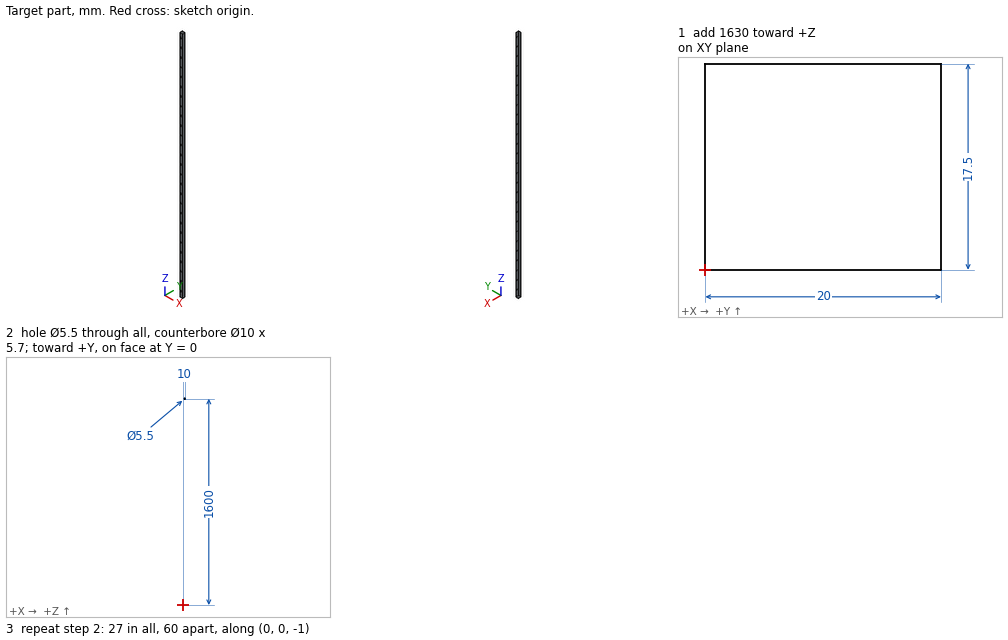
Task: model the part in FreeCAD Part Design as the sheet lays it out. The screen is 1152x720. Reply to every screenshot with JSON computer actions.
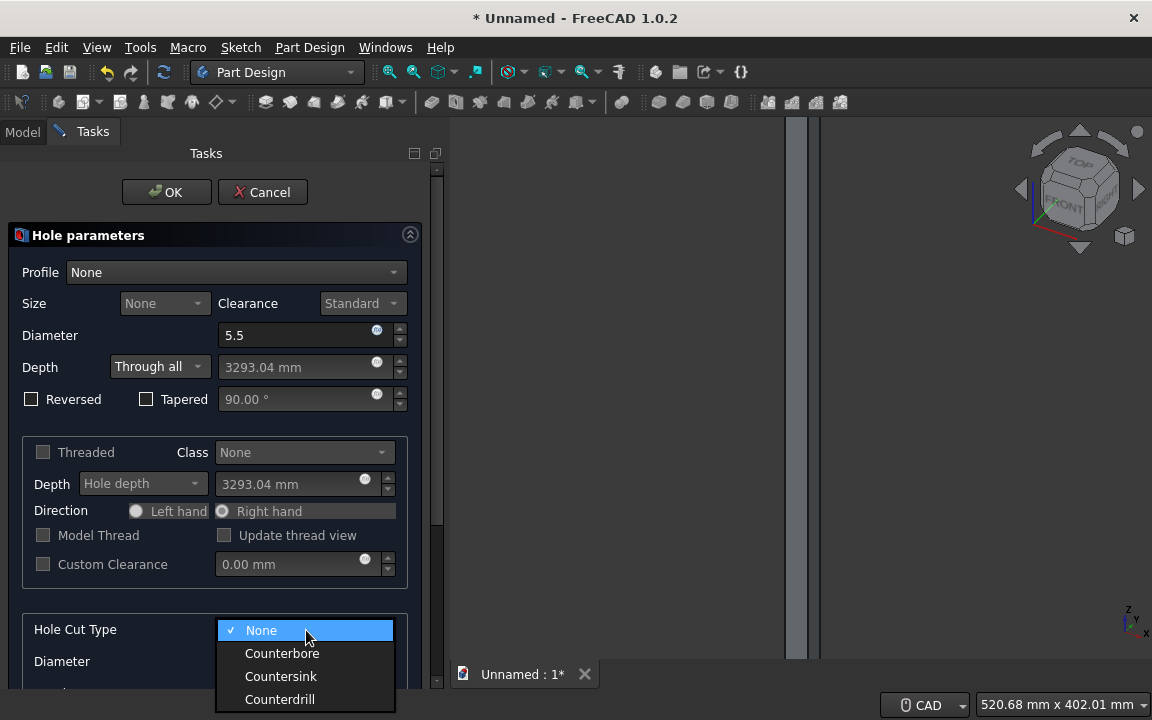
{"action": "left_click", "coordinate": [304, 654]}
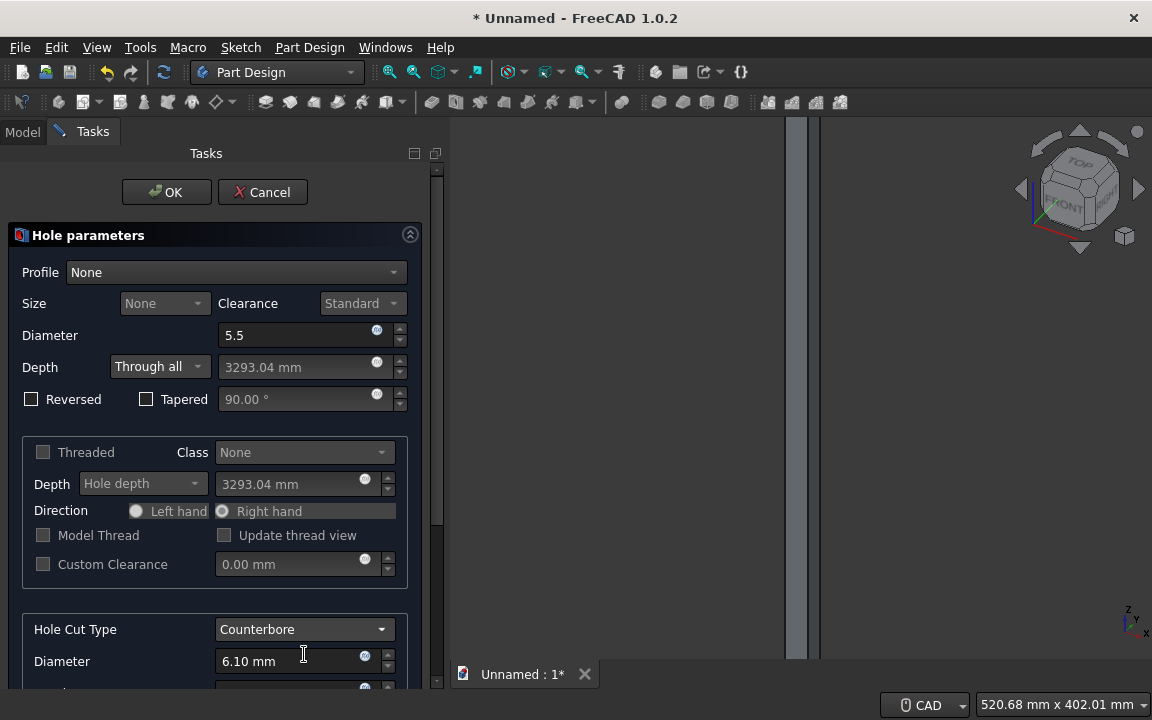
{"action": "triple_click", "coordinate": [298, 661]}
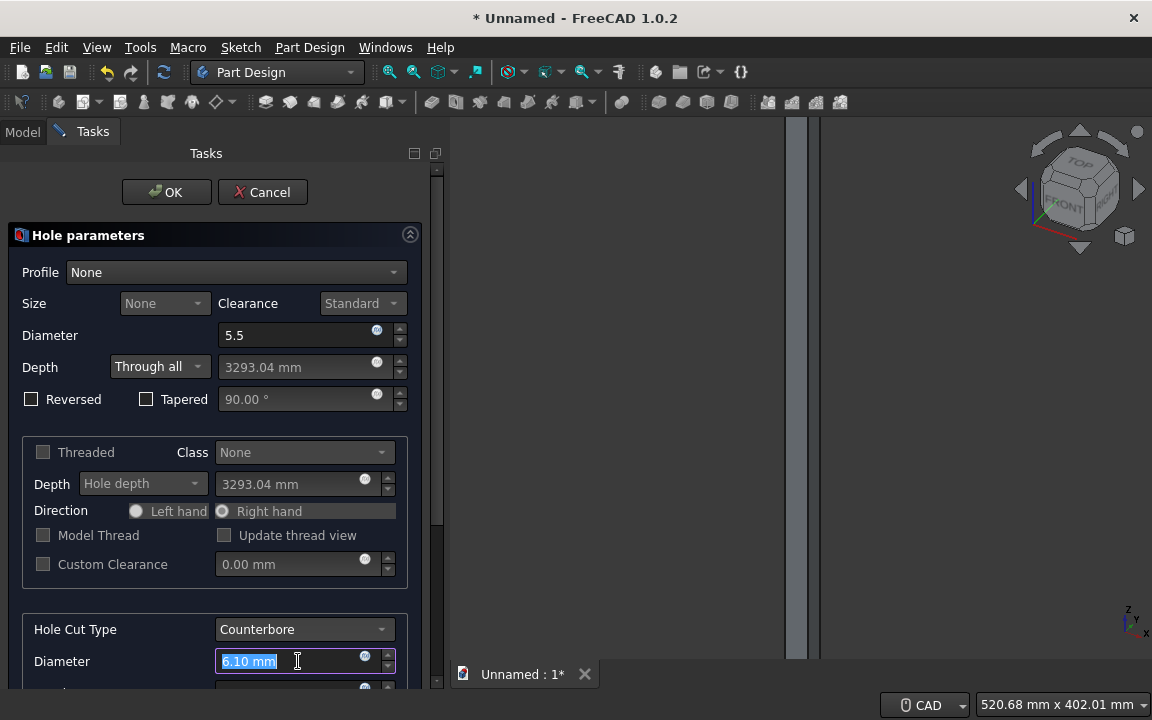
{"action": "type", "text": "10"}
{"action": "key", "text": "Tab"}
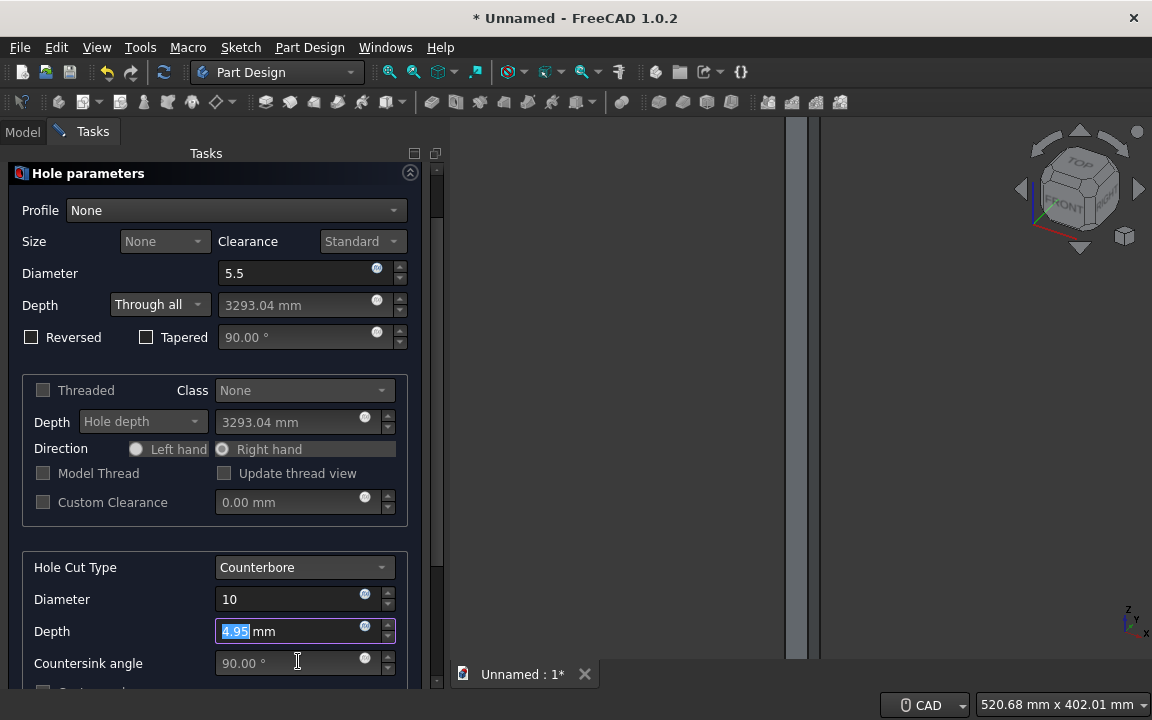
{"action": "type", "text": "5.7"}
{"action": "key", "text": "Tab"}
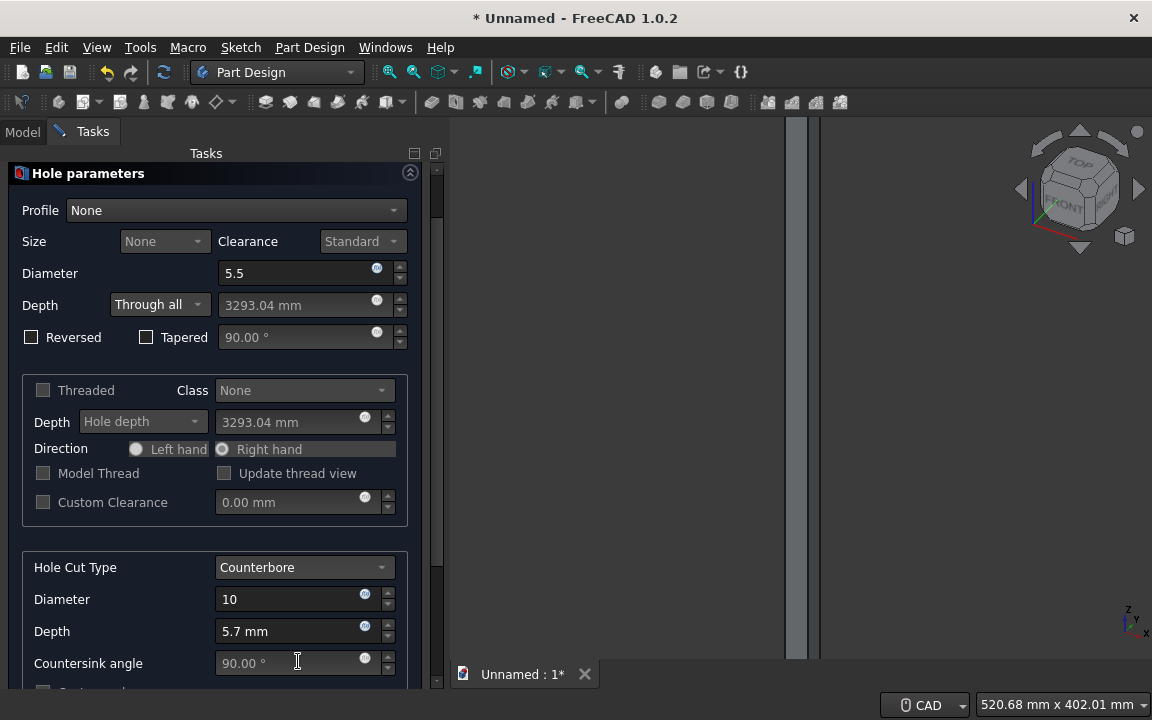
{"action": "scroll", "coordinate": [437, 426], "scroll_direction": "up", "scroll_amount": 2}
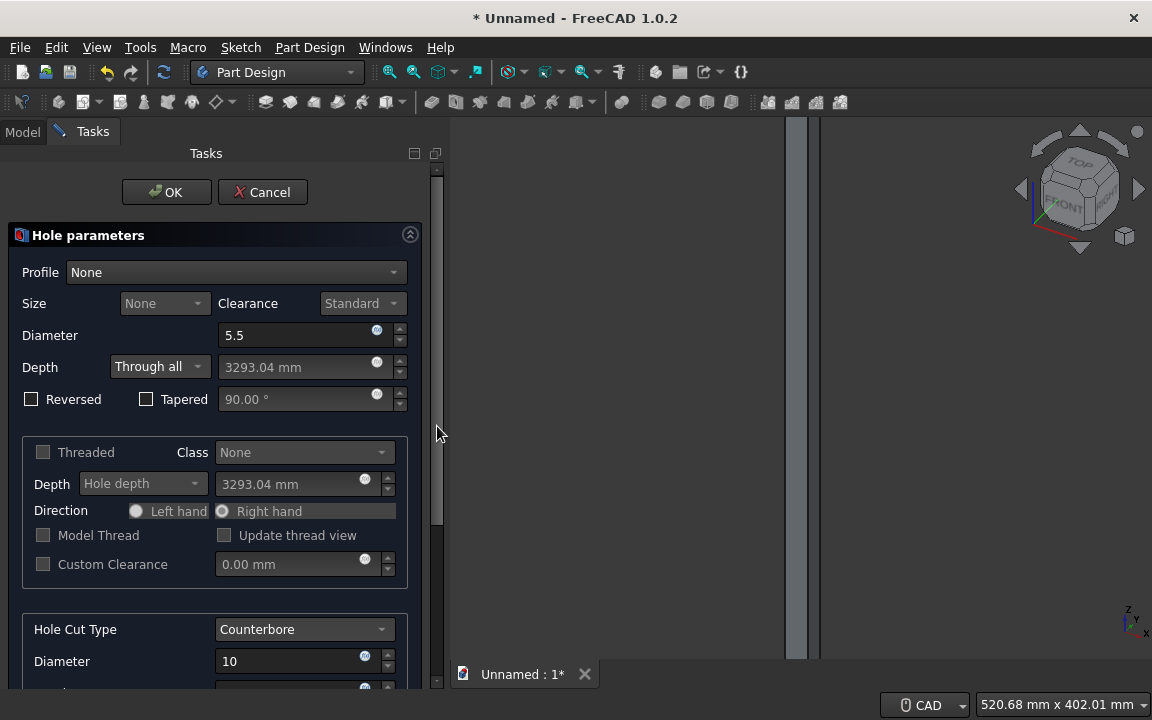
{"action": "left_click", "coordinate": [167, 192]}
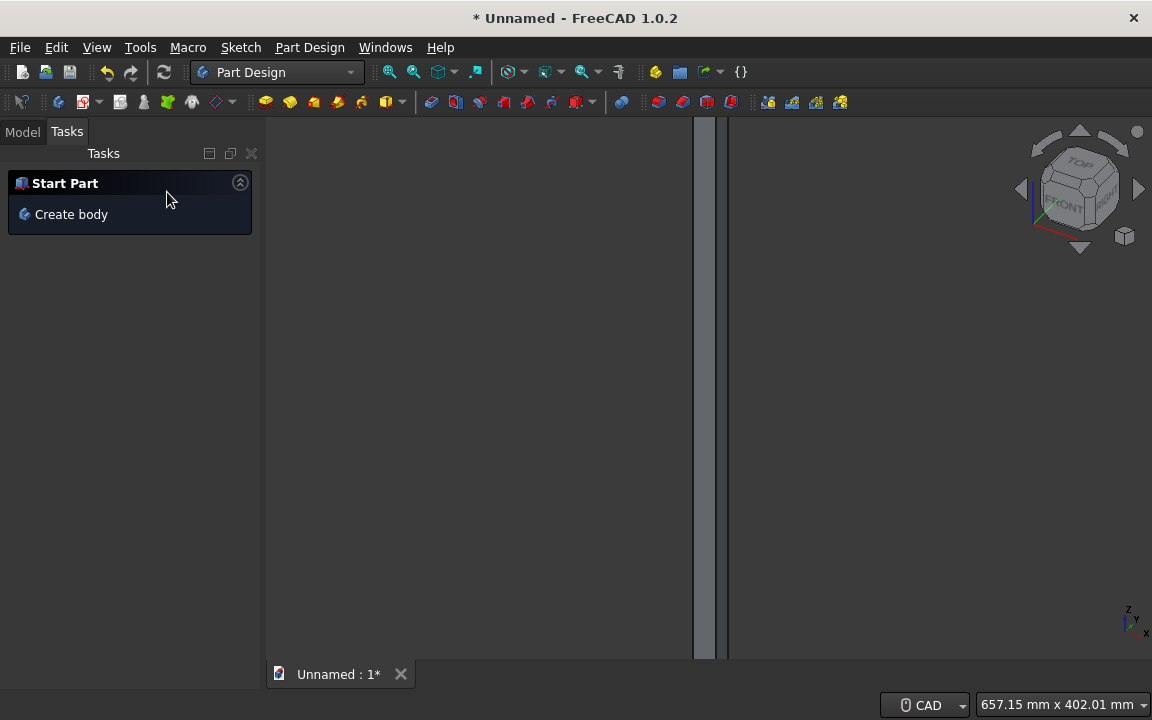
{"action": "left_click", "coordinate": [390, 72]}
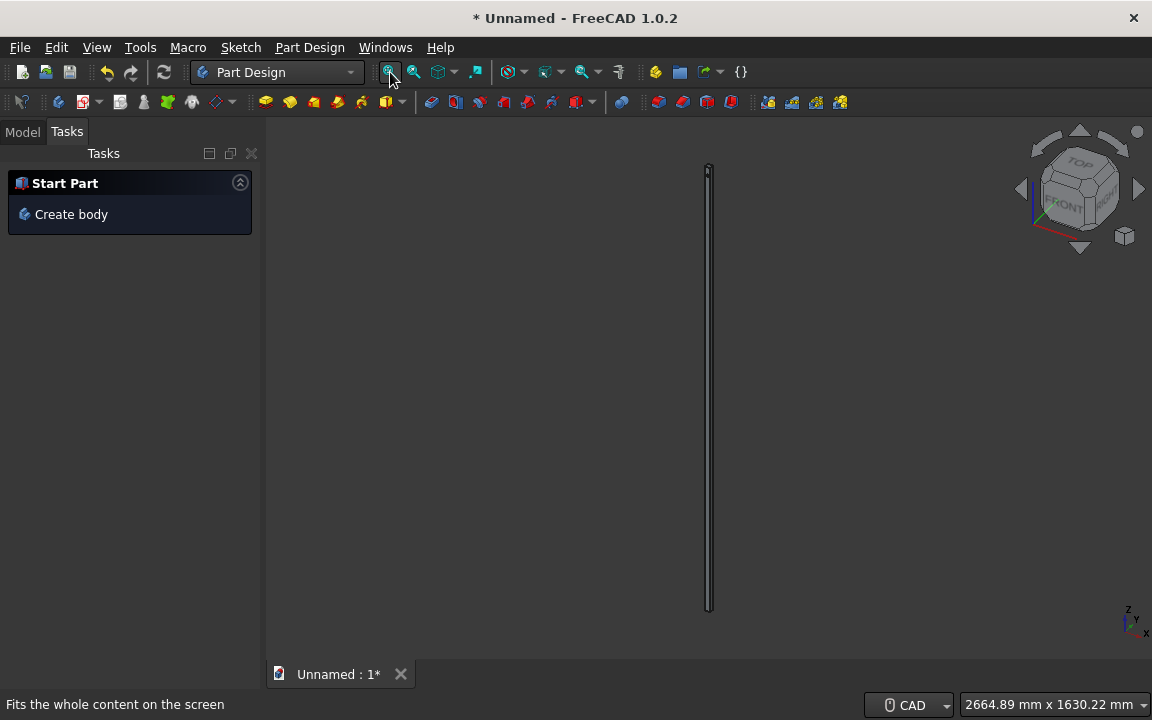
{"action": "left_click", "coordinate": [23, 131]}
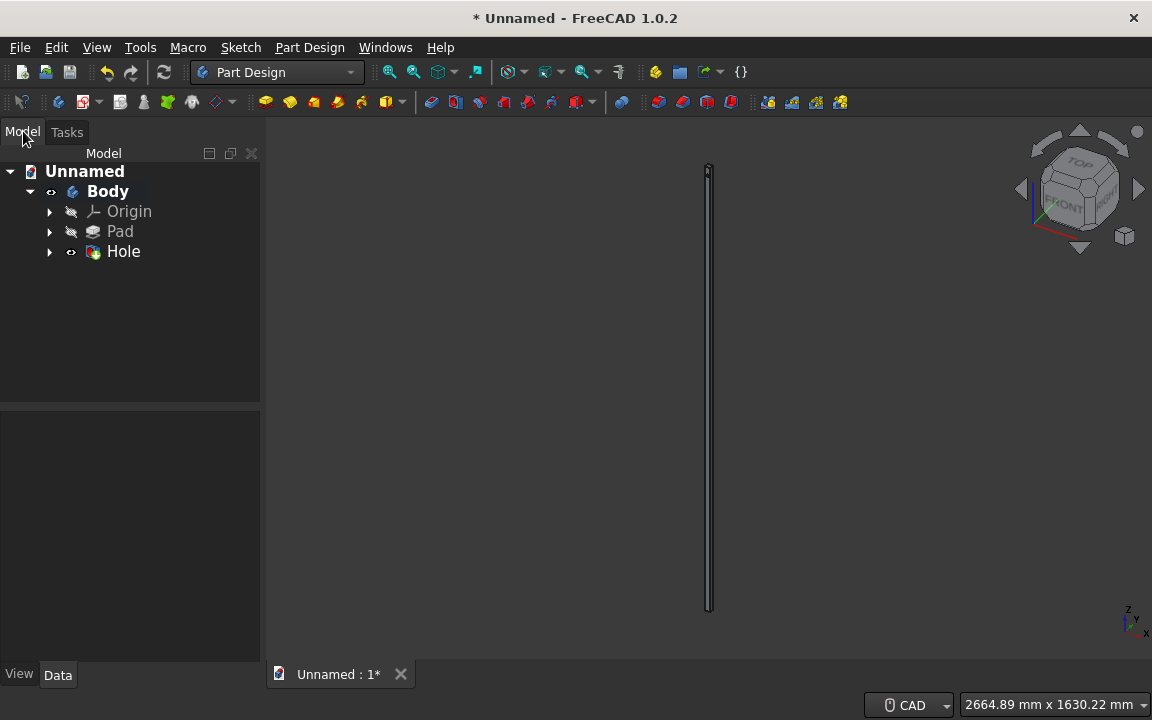
{"action": "left_click", "coordinate": [116, 252]}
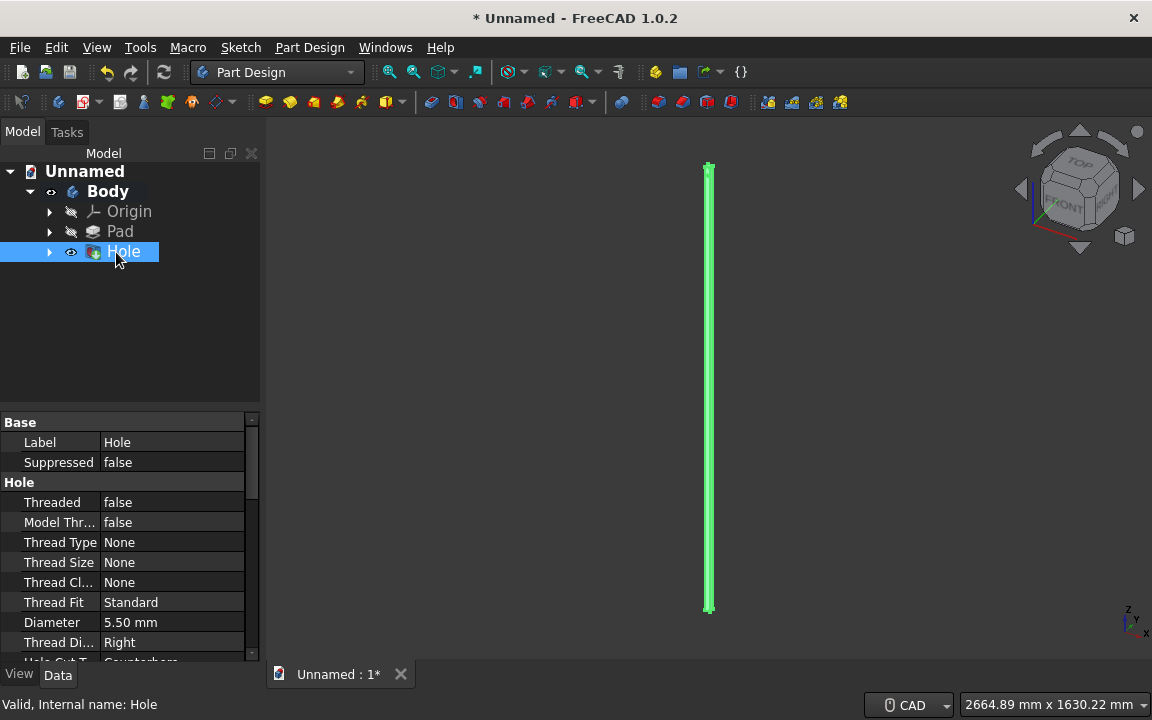
{"action": "left_click", "coordinate": [792, 102]}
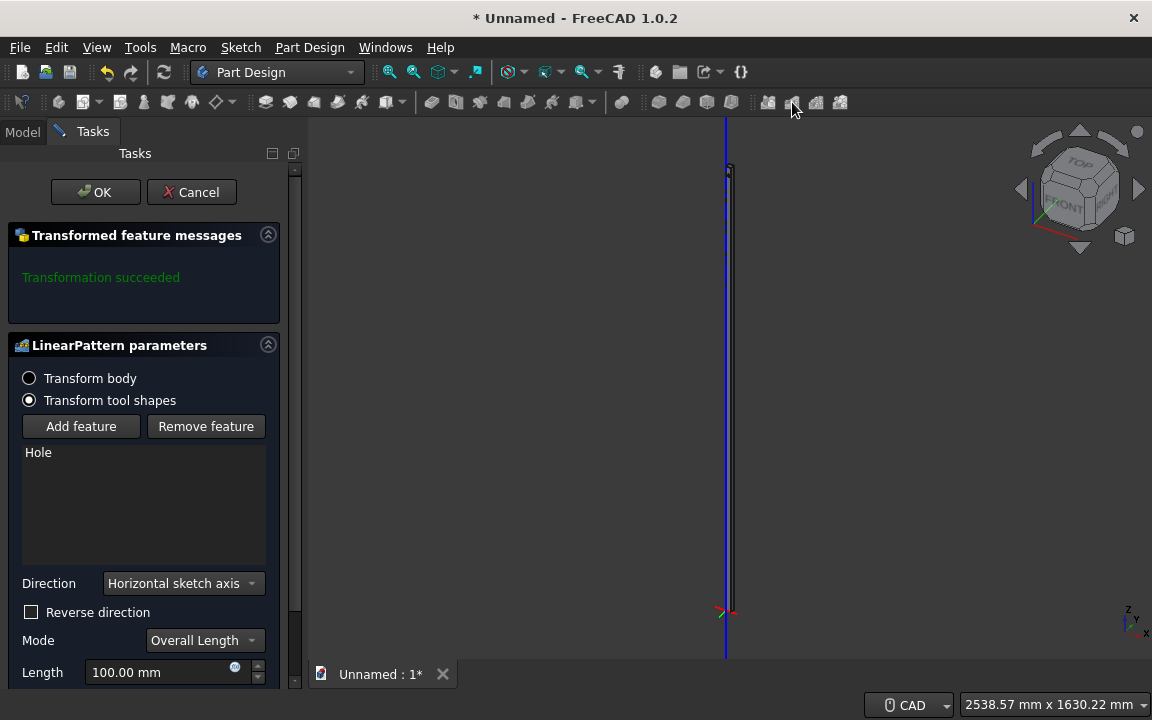
{"action": "left_click", "coordinate": [184, 584]}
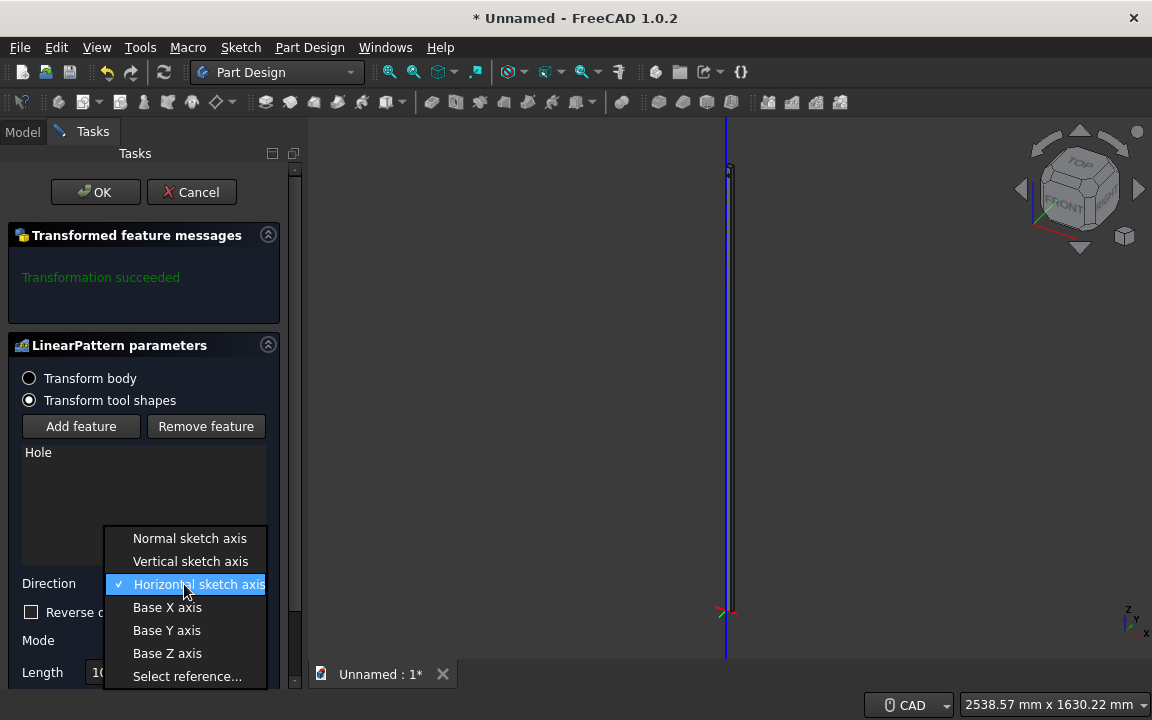
{"action": "left_click", "coordinate": [184, 654]}